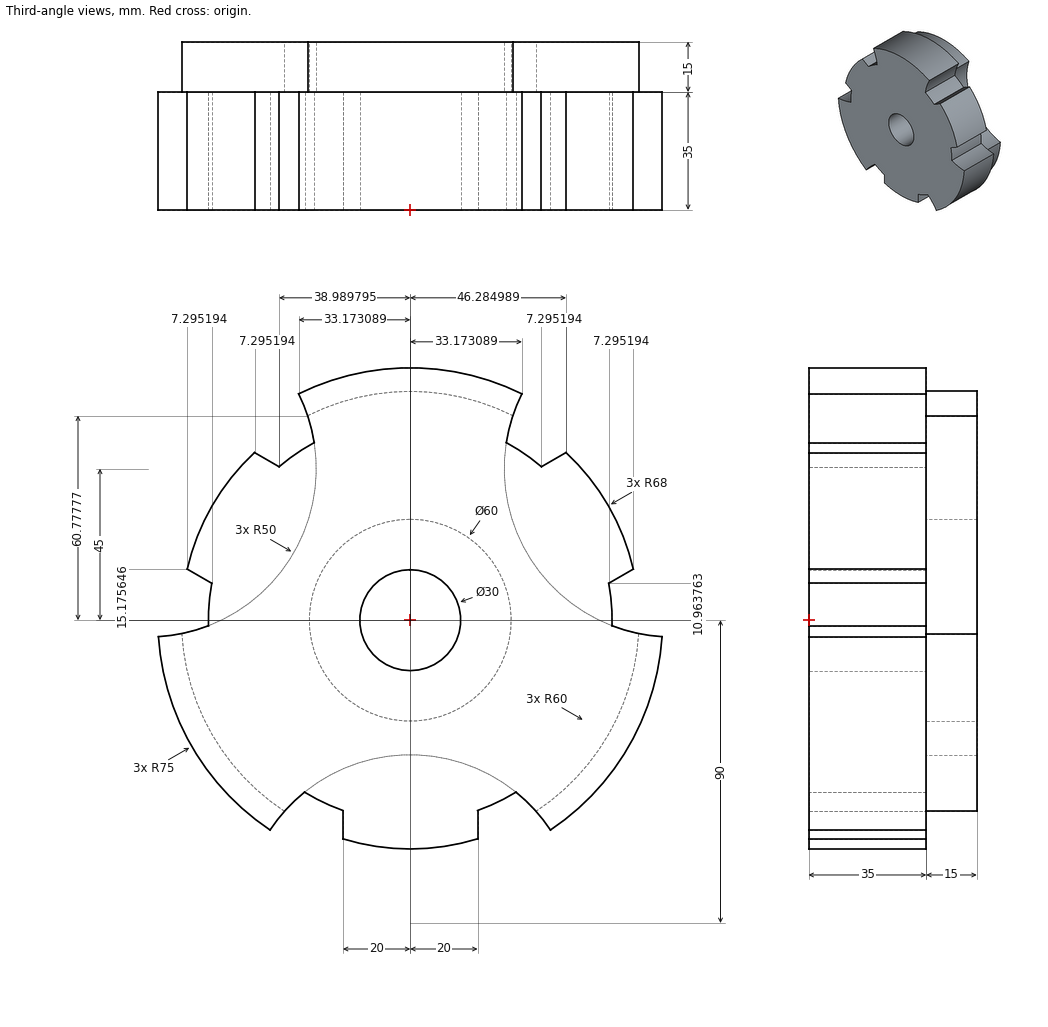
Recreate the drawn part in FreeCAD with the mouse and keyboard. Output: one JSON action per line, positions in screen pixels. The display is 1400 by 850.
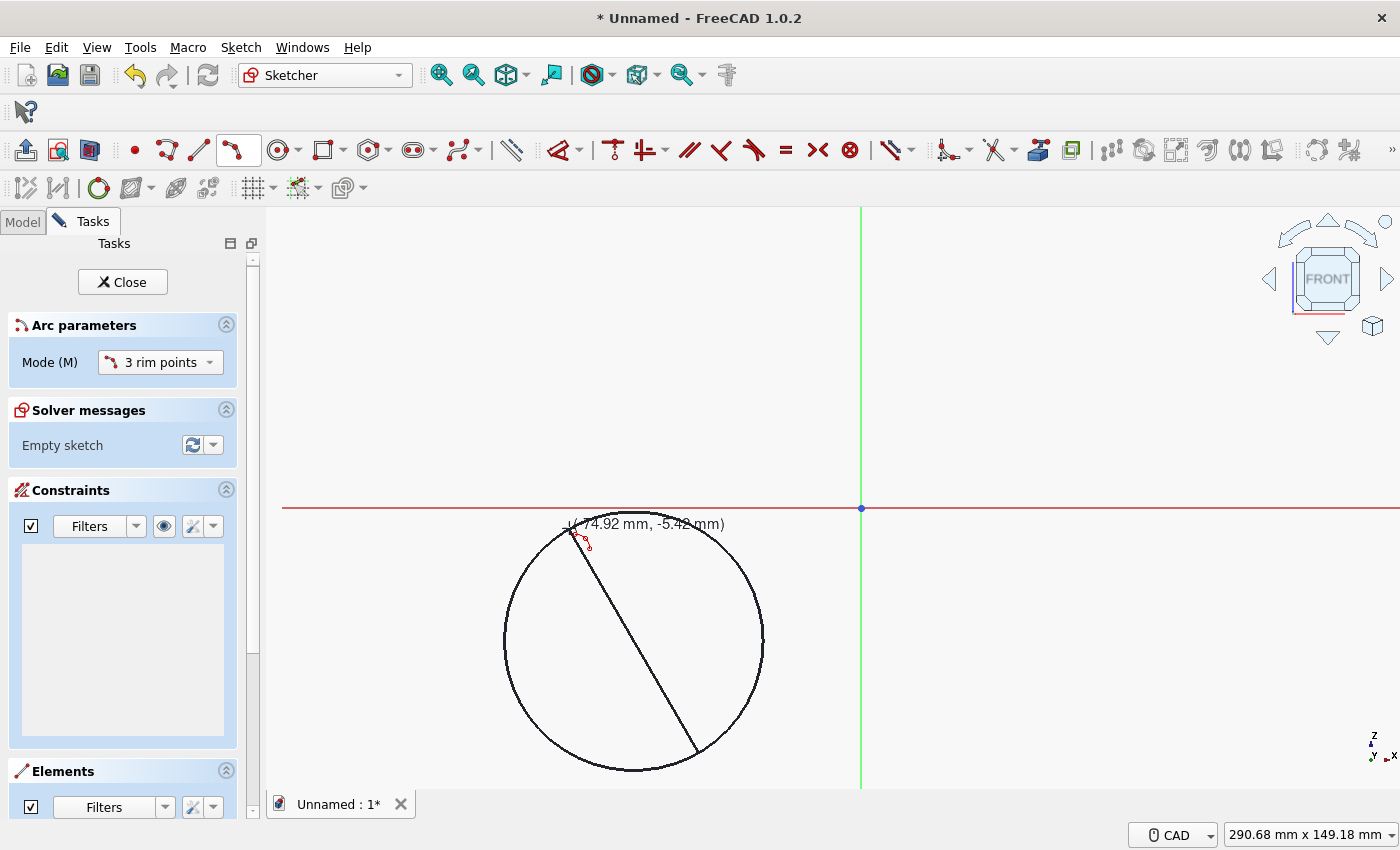
{"action": "left_click", "coordinate": [569, 527]}
{"action": "left_click", "coordinate": [608, 654]}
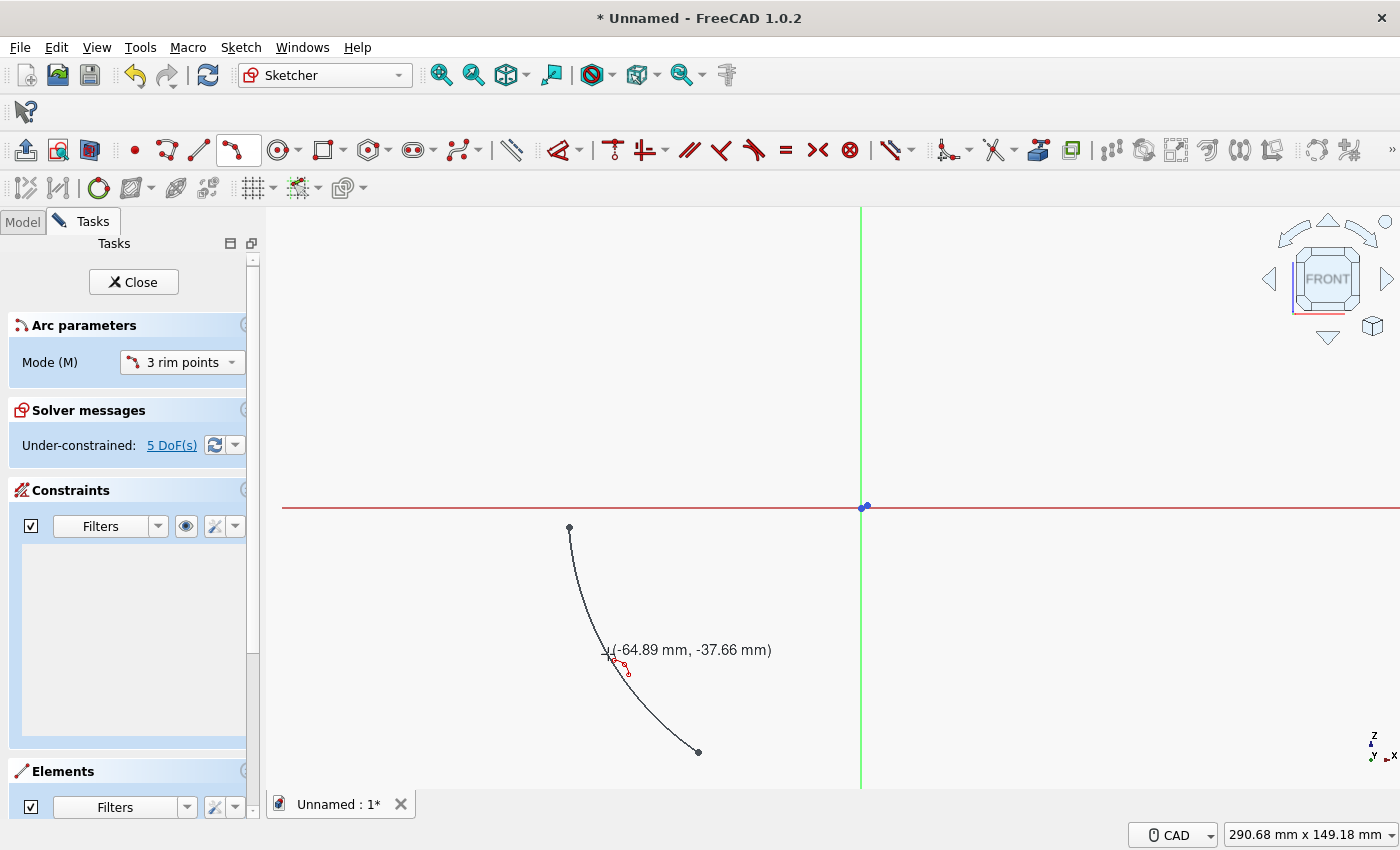
{"action": "left_click", "coordinate": [569, 528]}
{"action": "left_click", "coordinate": [732, 246]}
{"action": "left_click", "coordinate": [726, 430]}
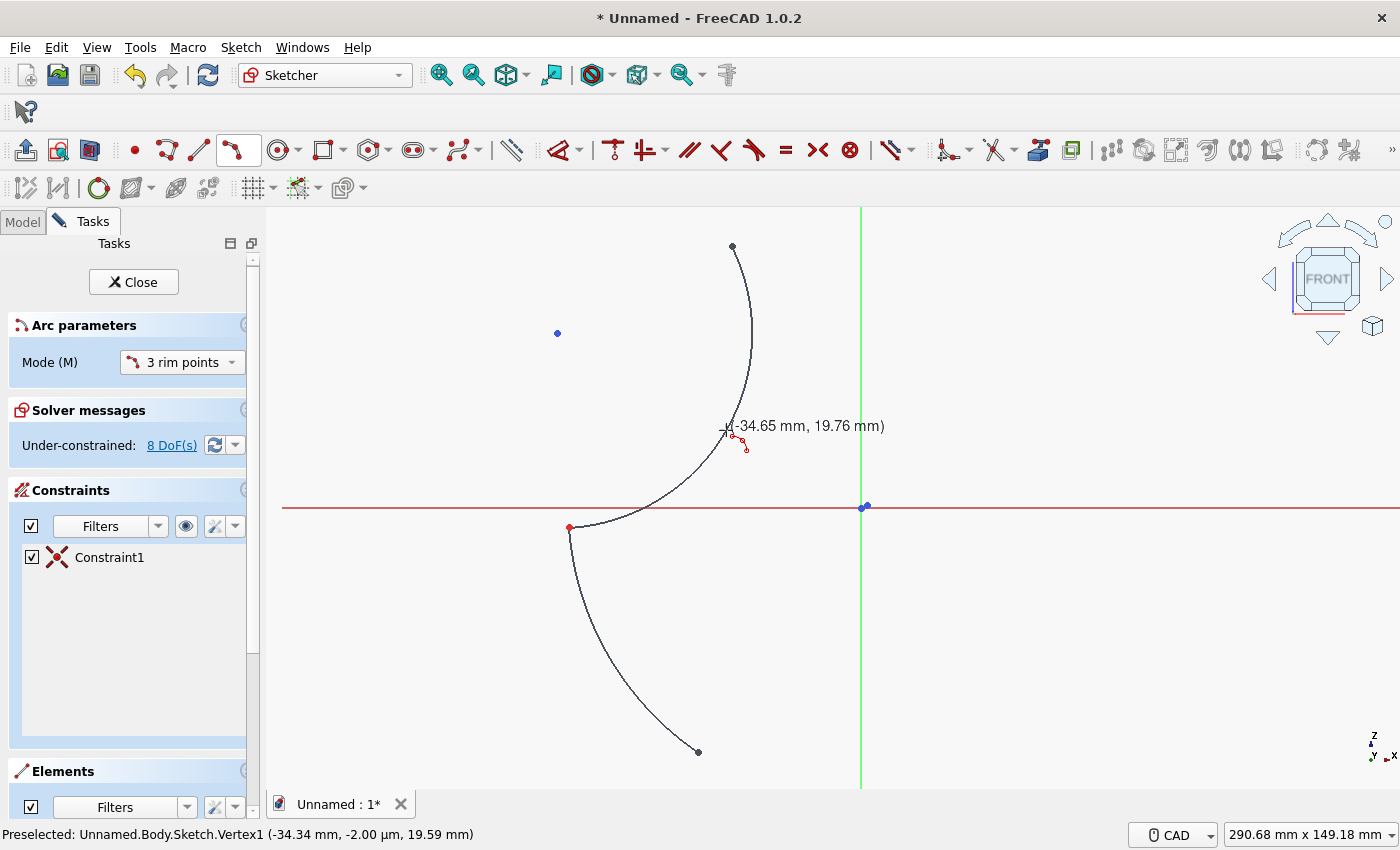
{"action": "left_click", "coordinate": [732, 247]}
{"action": "left_click", "coordinate": [991, 246]}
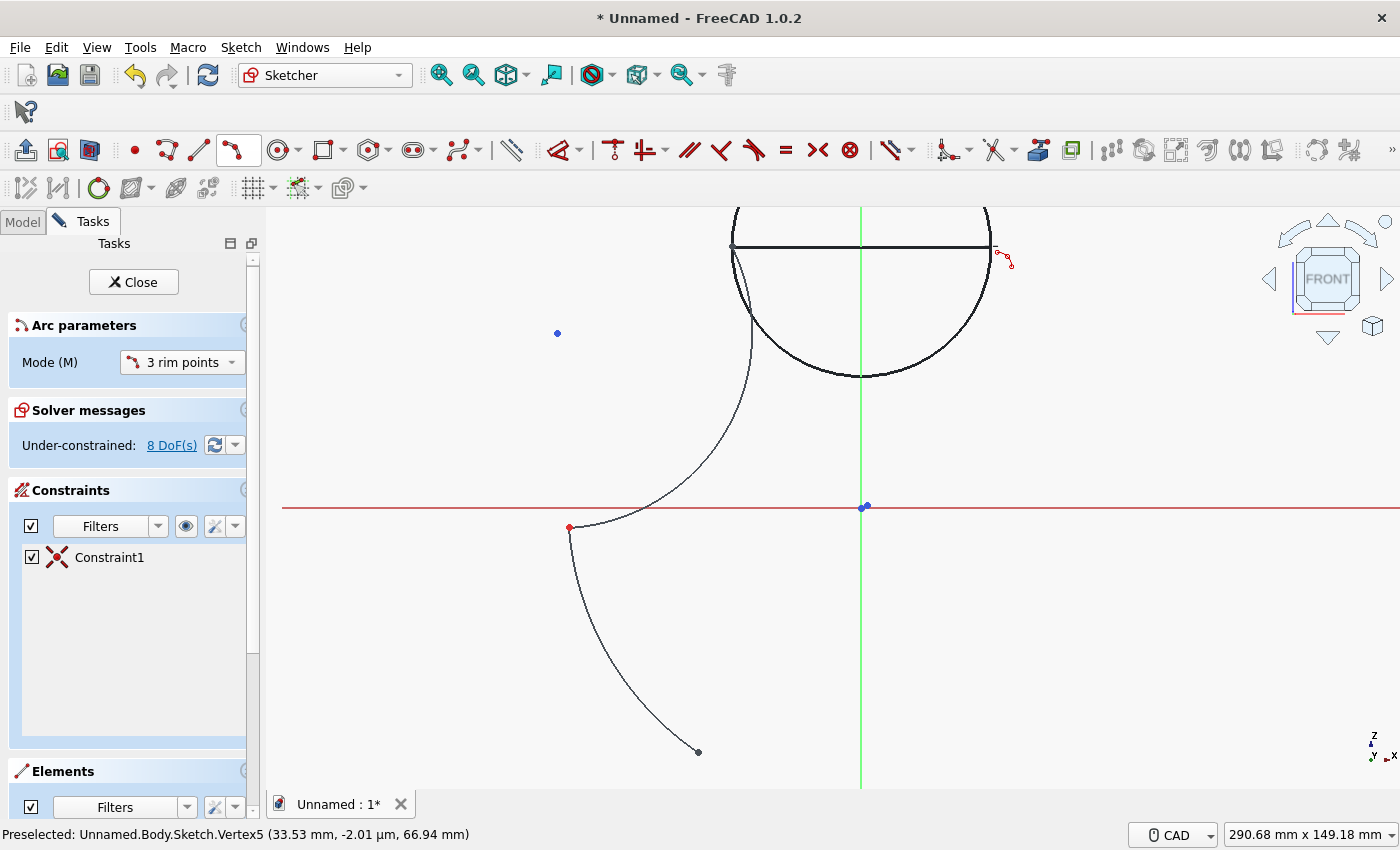
{"action": "scroll", "coordinate": [568, 528], "scroll_direction": "down", "scroll_amount": 2}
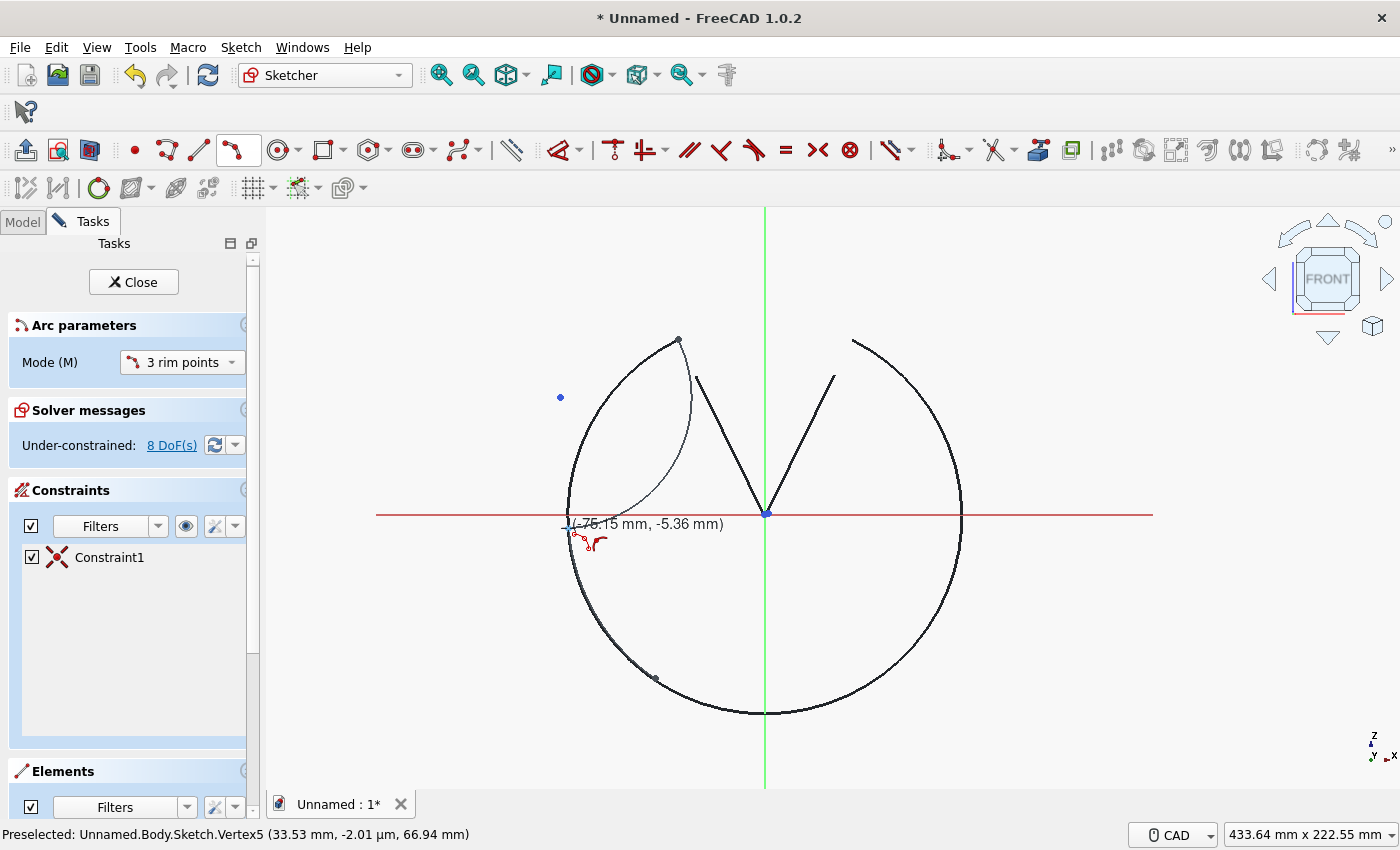
{"action": "left_click", "coordinate": [783, 320]}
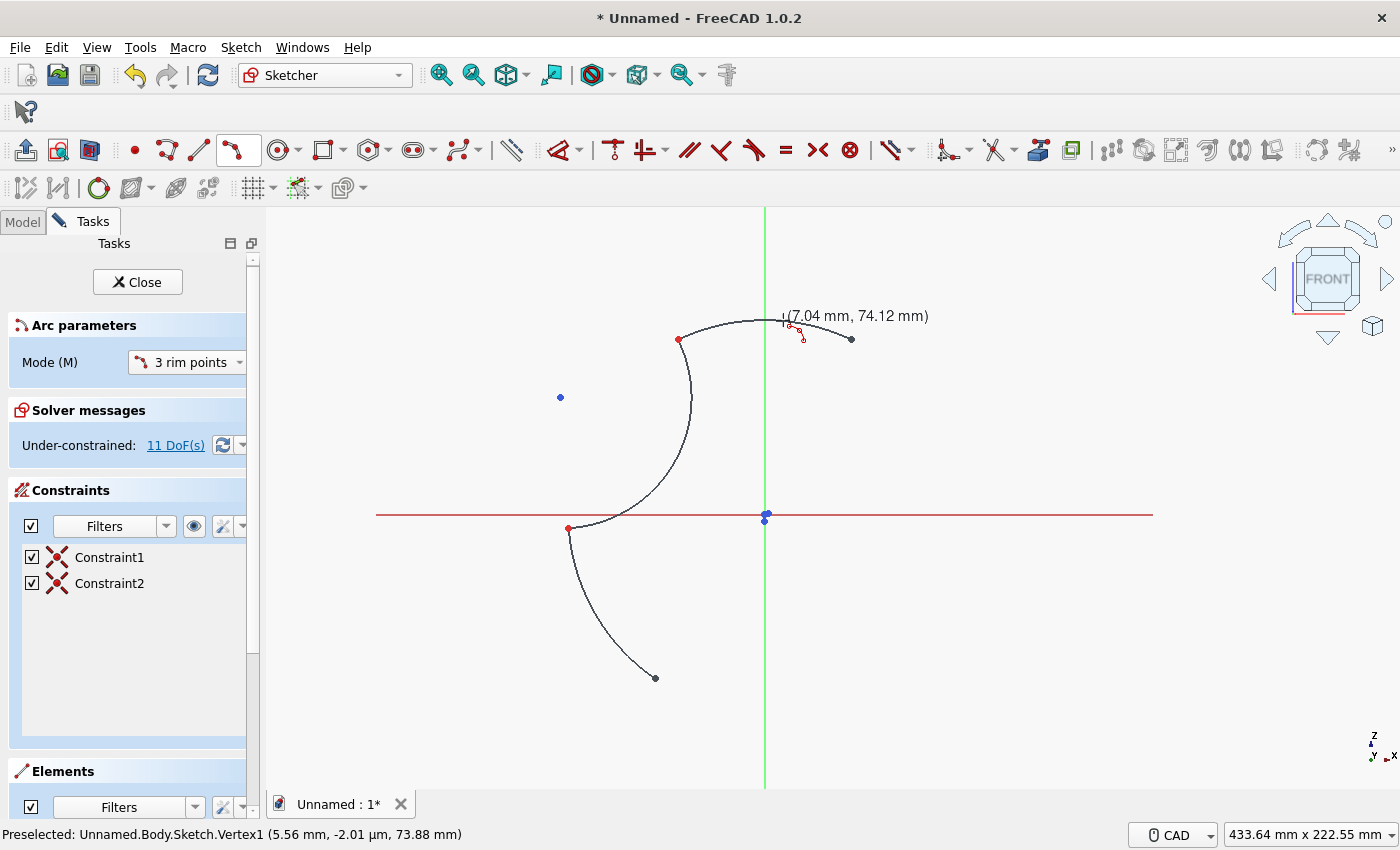
{"action": "left_click", "coordinate": [852, 340]}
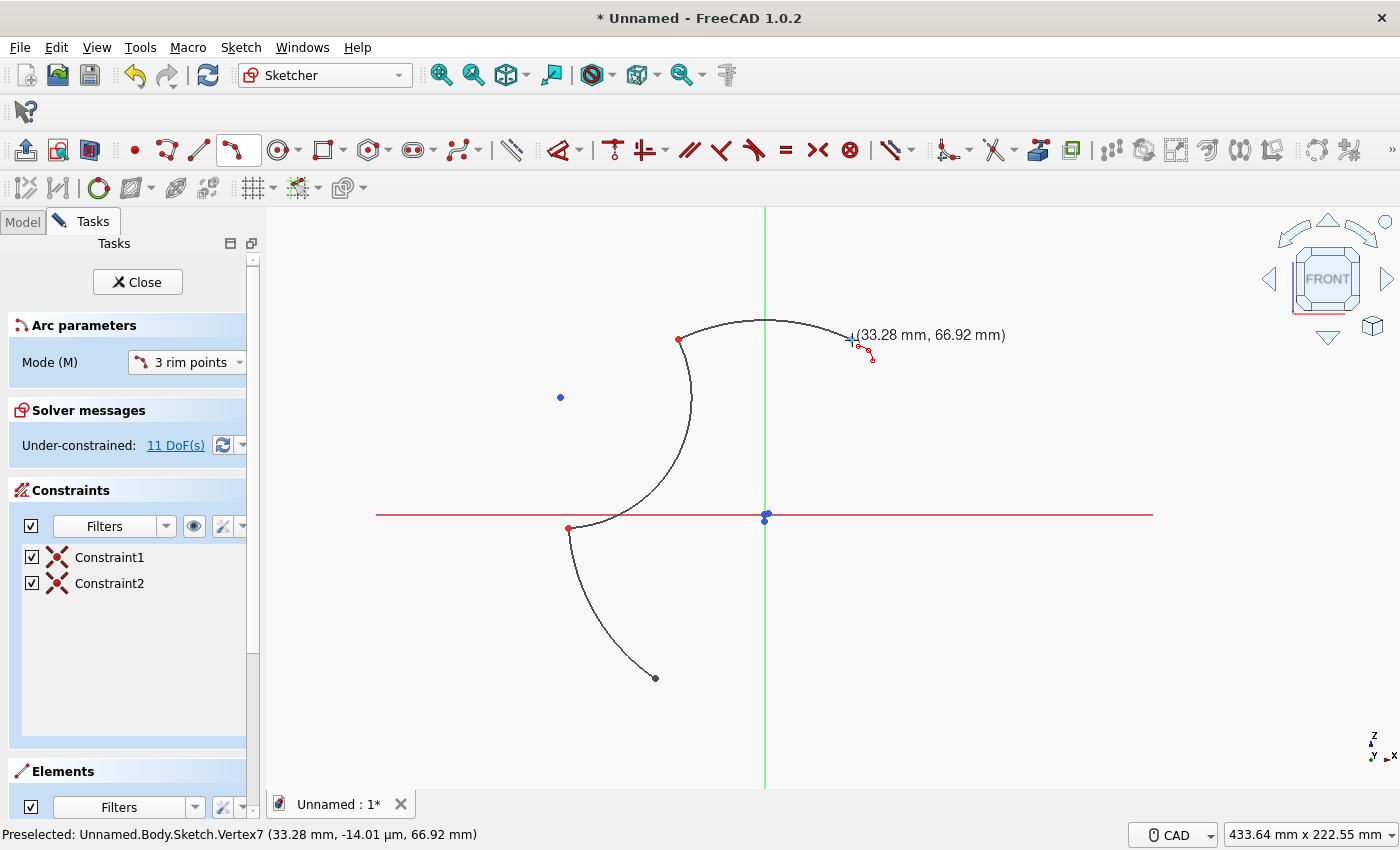
{"action": "scroll", "coordinate": [960, 528], "scroll_direction": "up", "scroll_amount": 2}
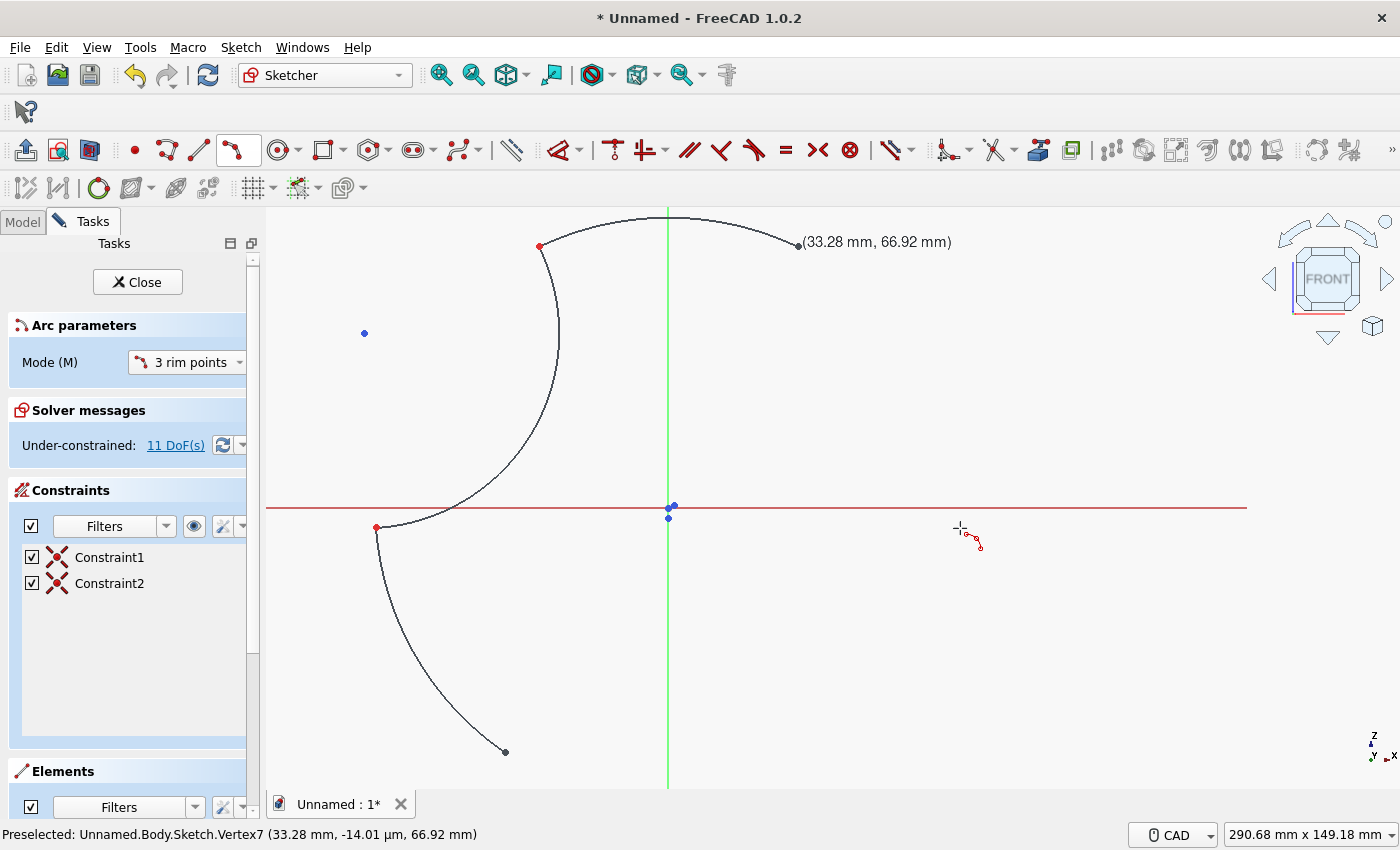
{"action": "left_click", "coordinate": [960, 527]}
{"action": "left_click", "coordinate": [803, 430]}